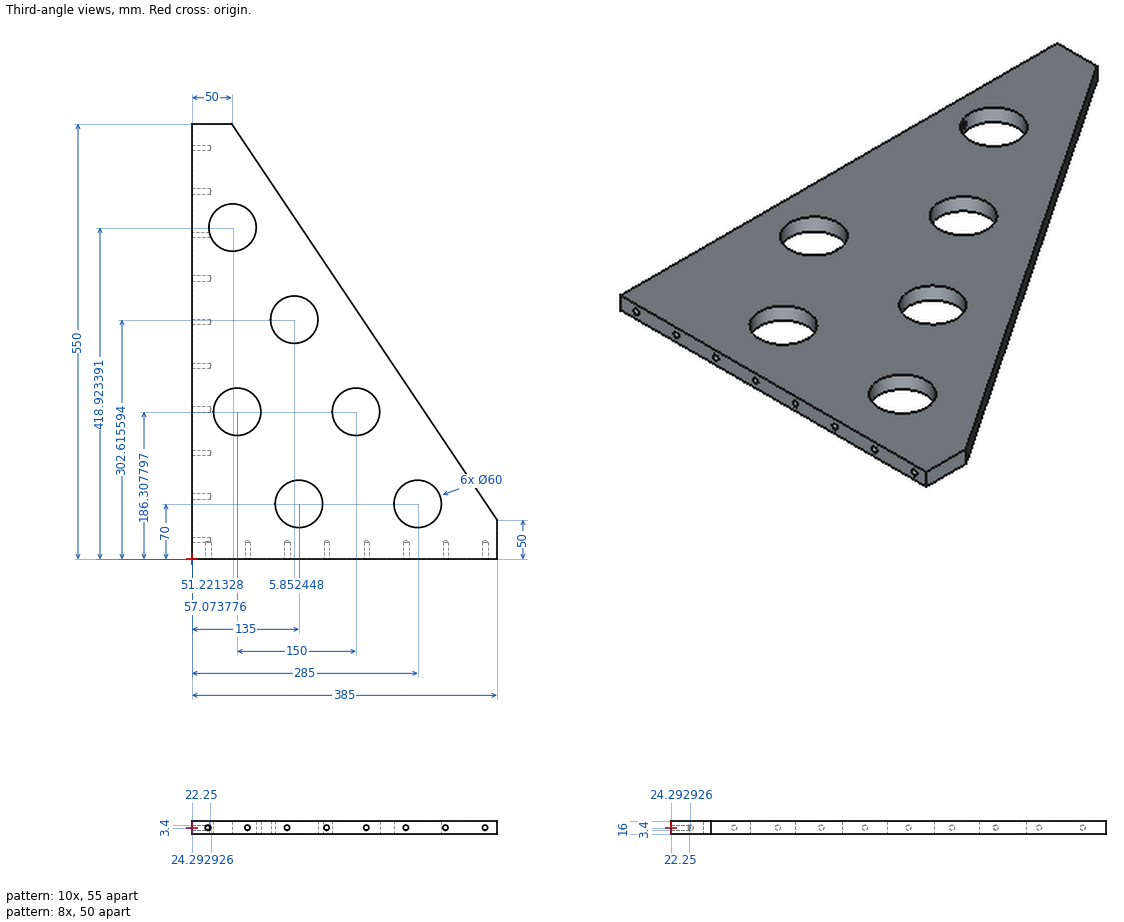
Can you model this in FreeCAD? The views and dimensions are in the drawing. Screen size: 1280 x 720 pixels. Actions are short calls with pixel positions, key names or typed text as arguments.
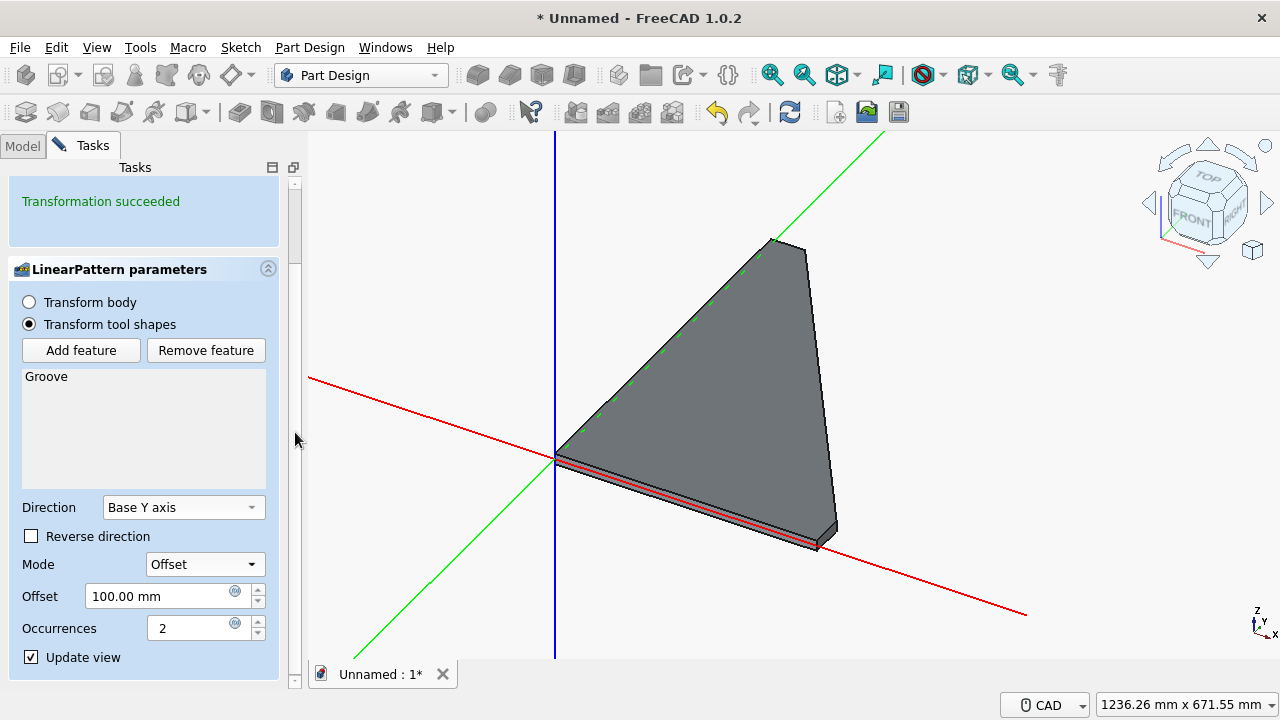
triple_click(168, 596)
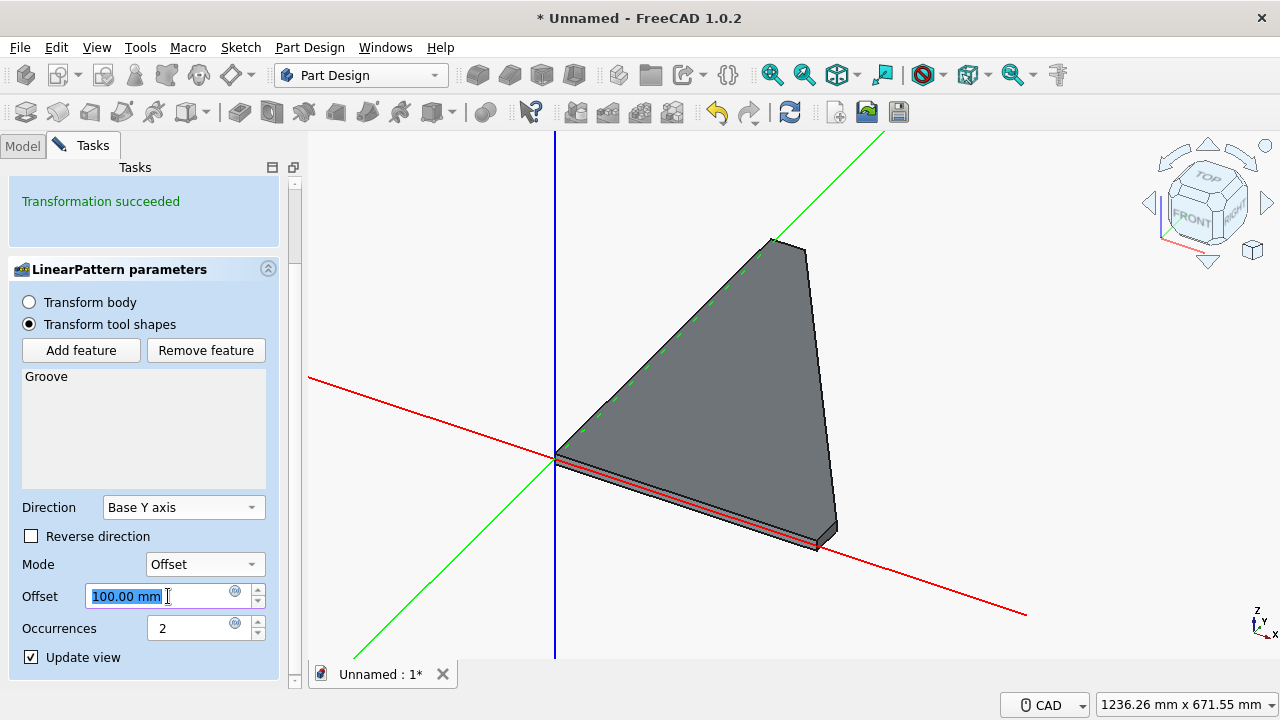
text(55)
key(Tab)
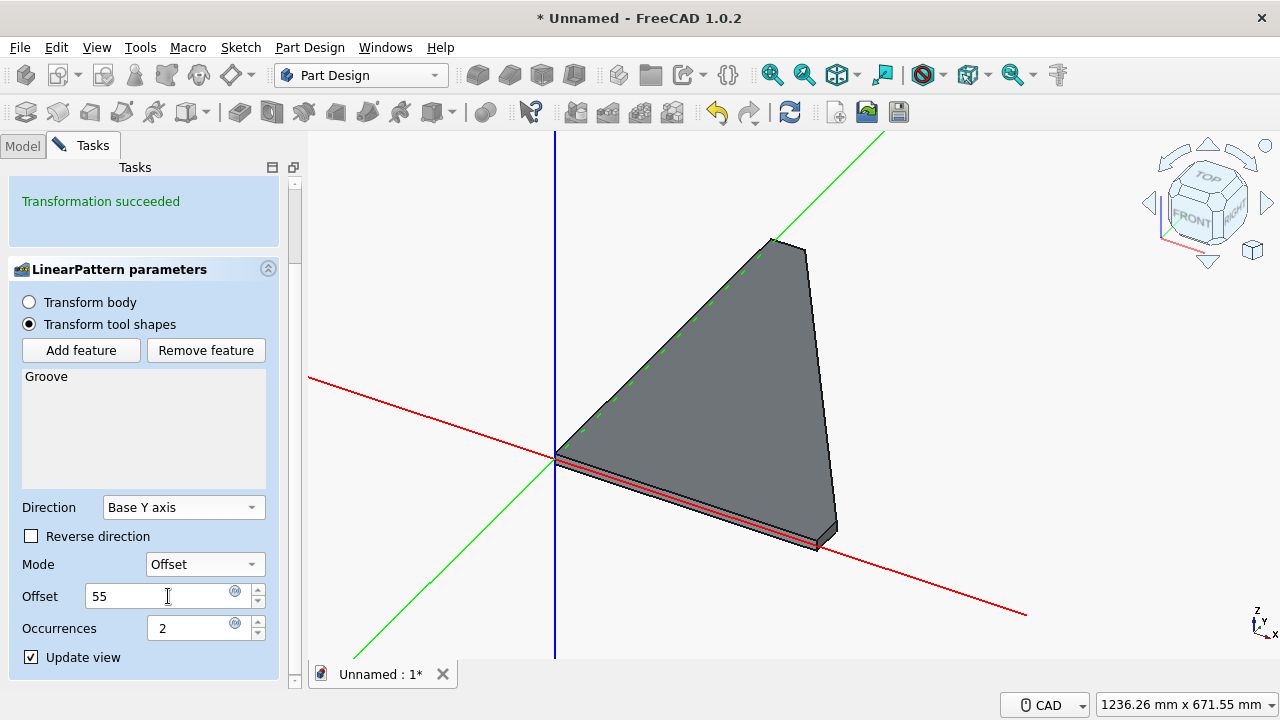
triple_click(198, 628)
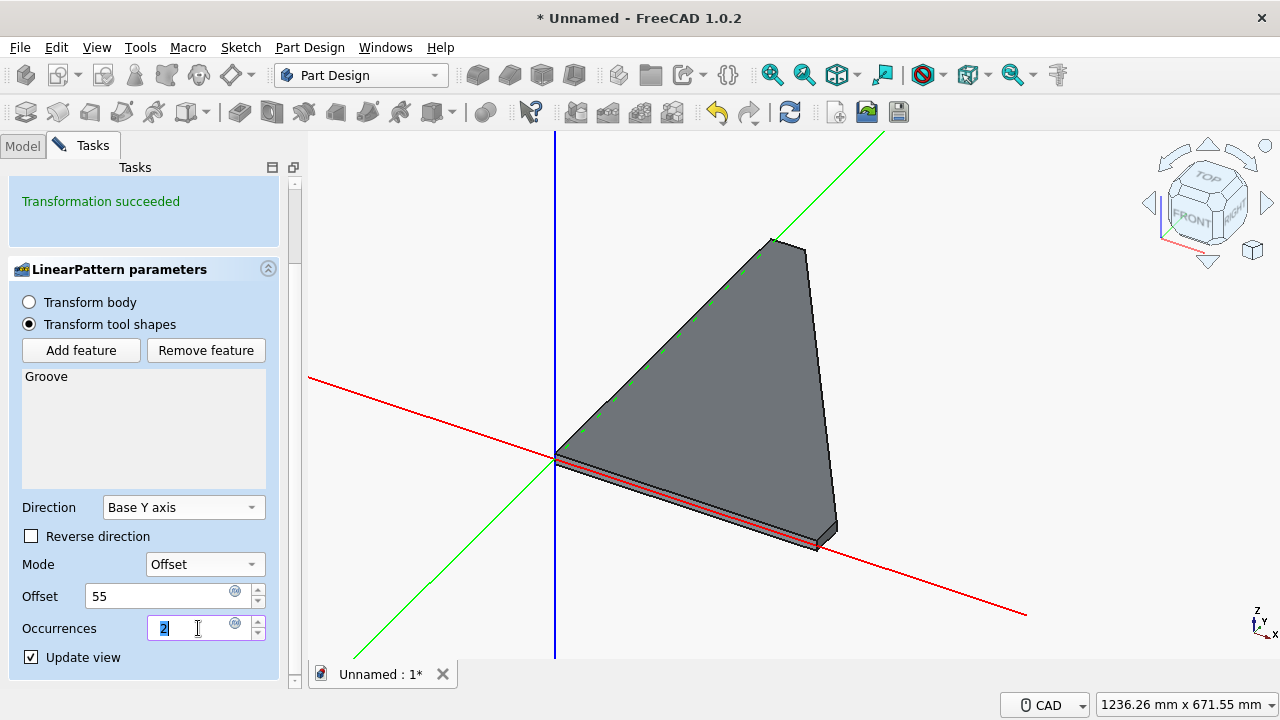
text(10)
key(Tab)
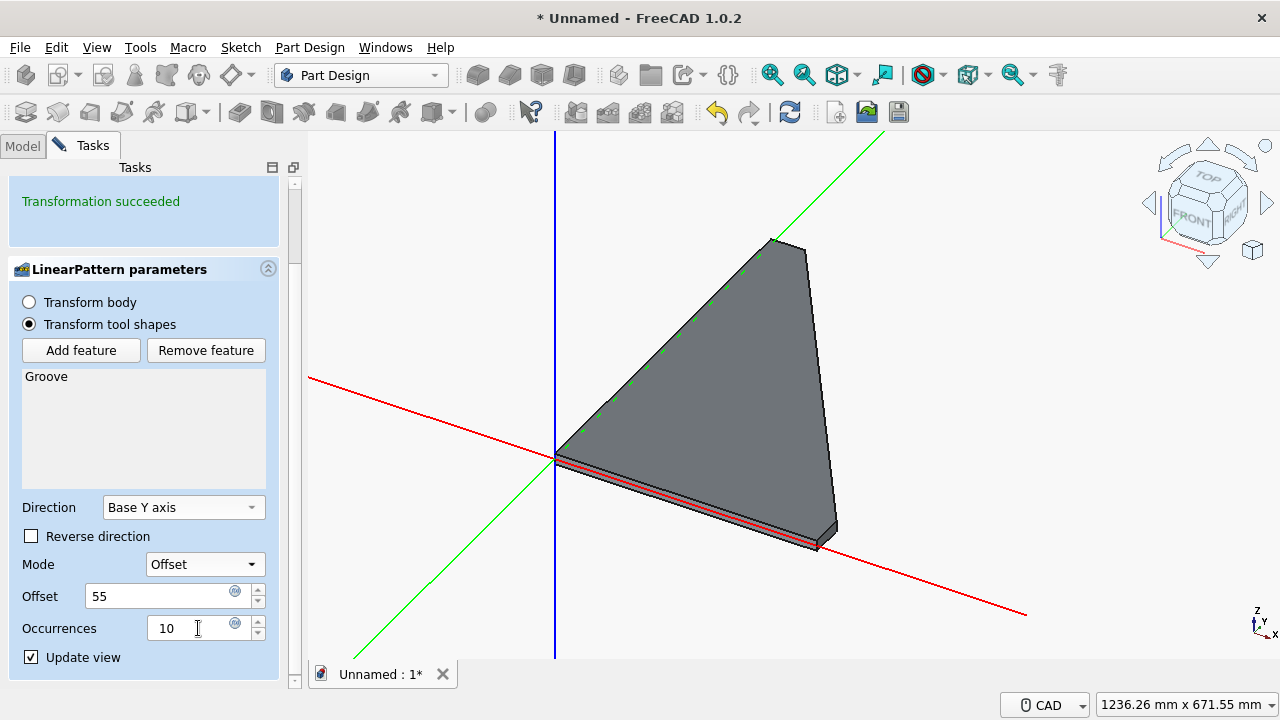
click(30, 536)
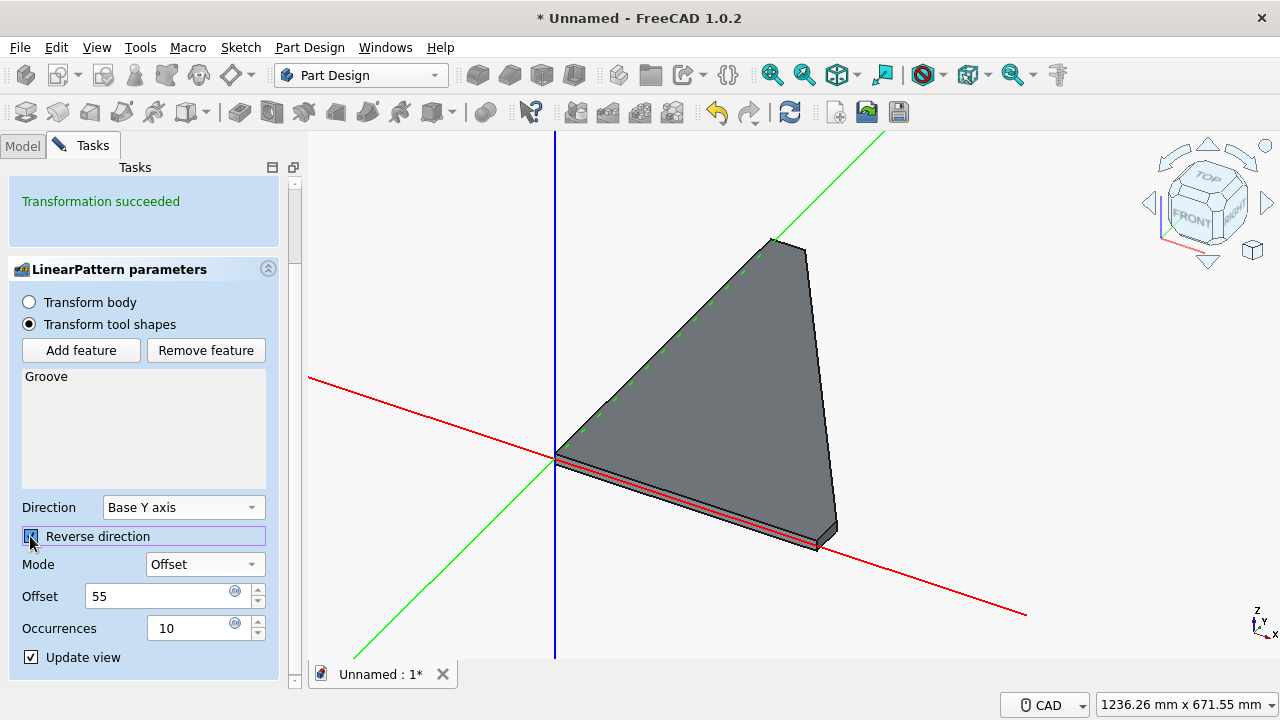
scroll(295, 432, up, 3)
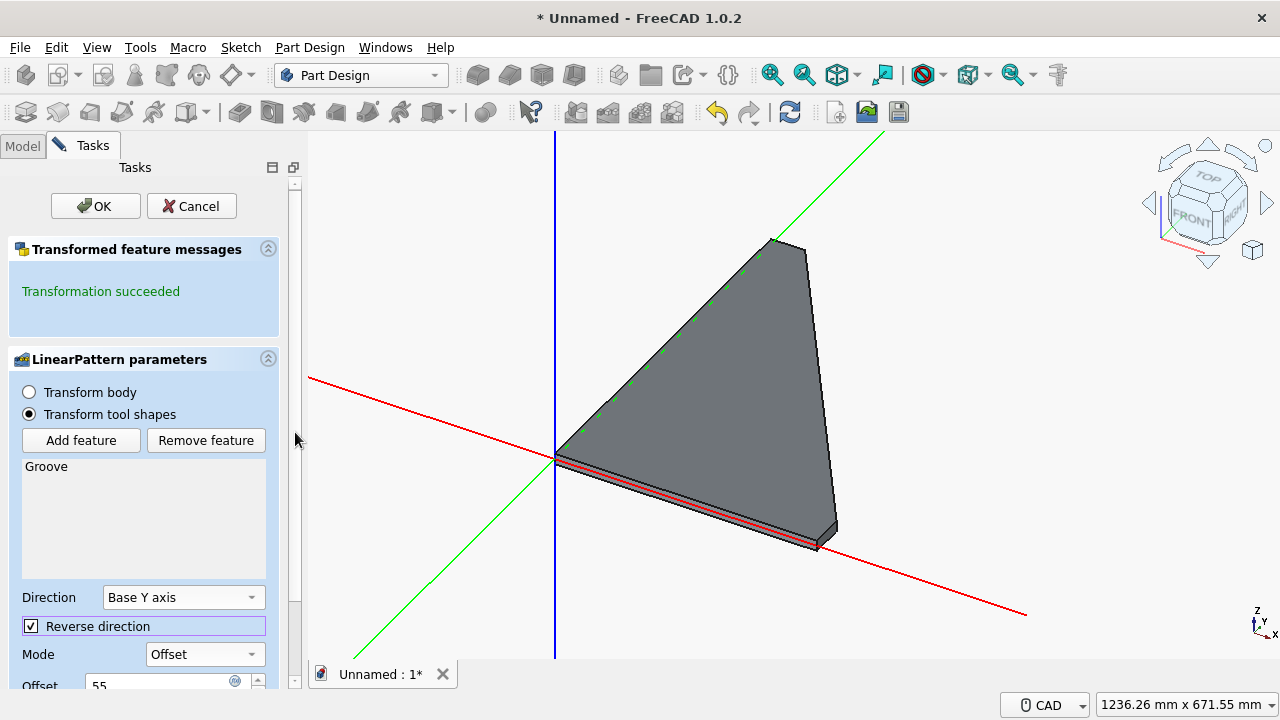
click(96, 206)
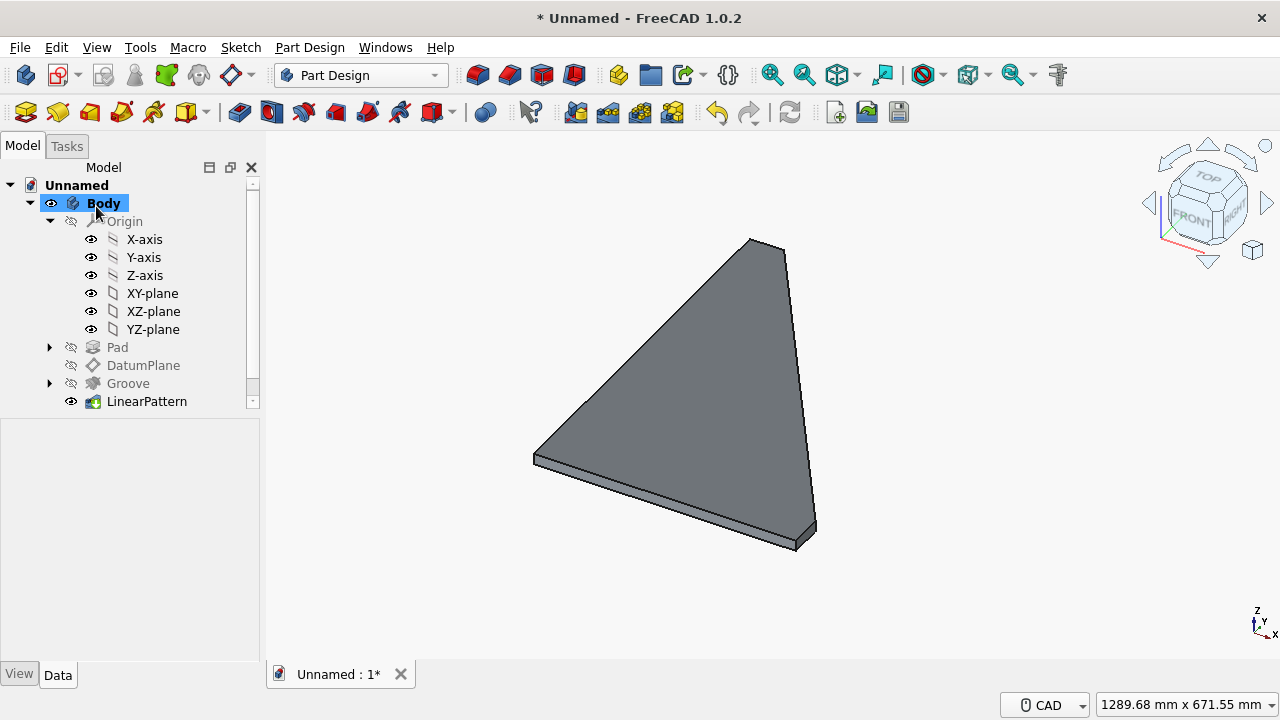
click(136, 329)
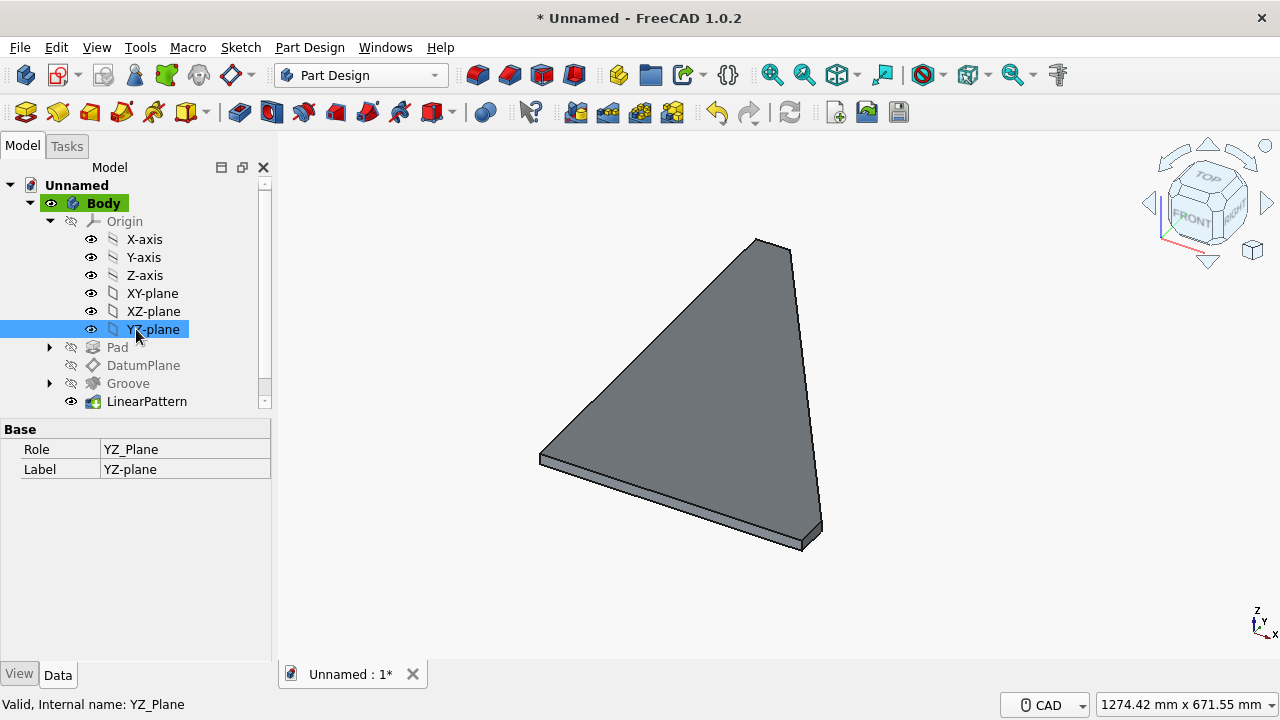
click(232, 76)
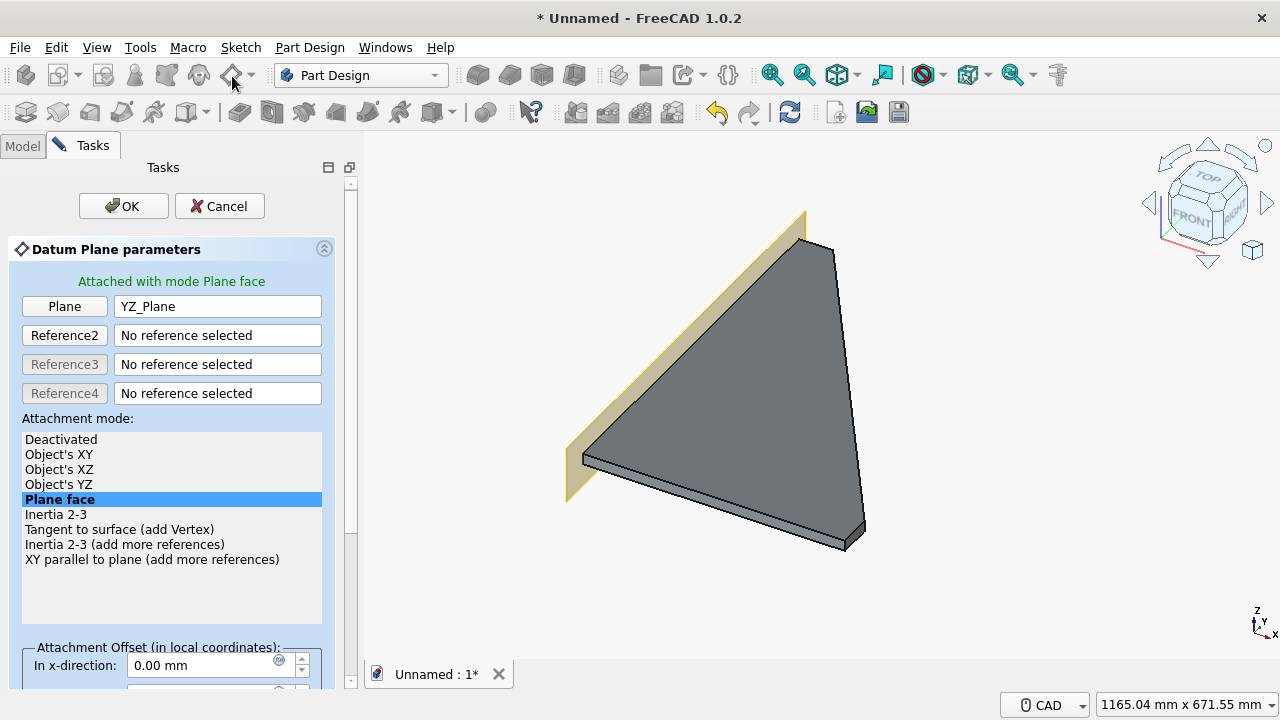
scroll(351, 432, down, 2)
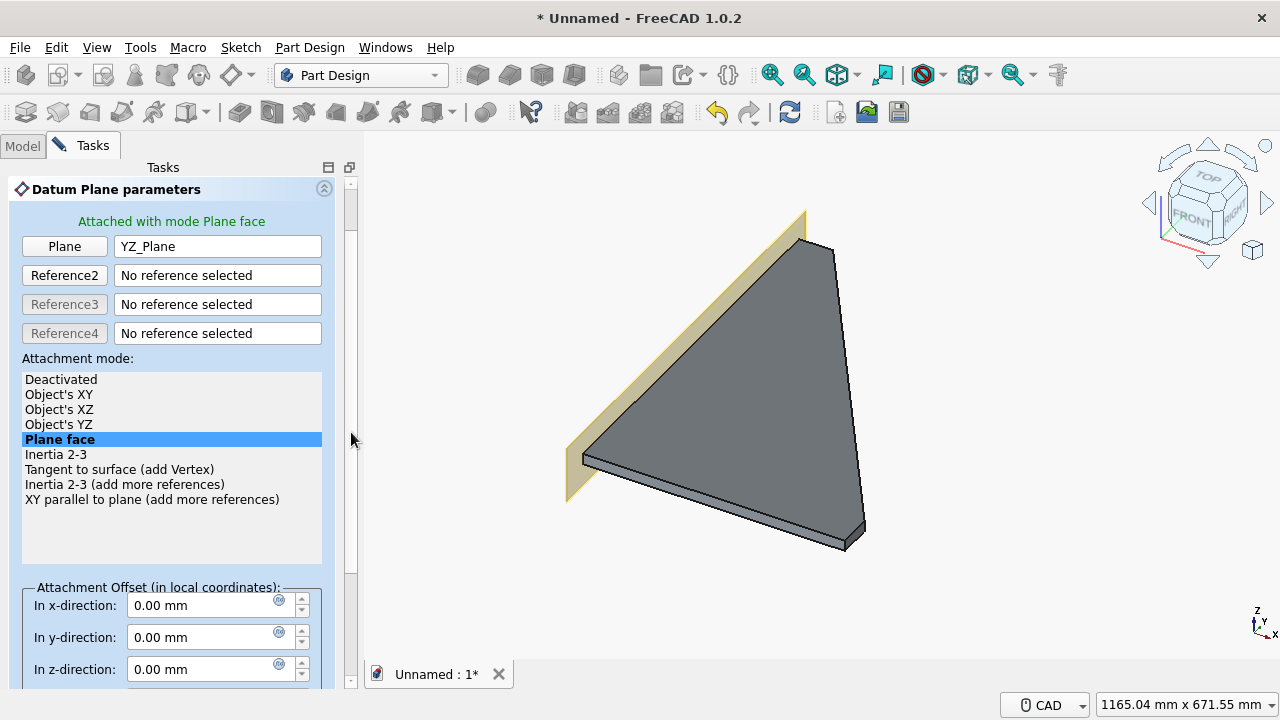
triple_click(210, 609)